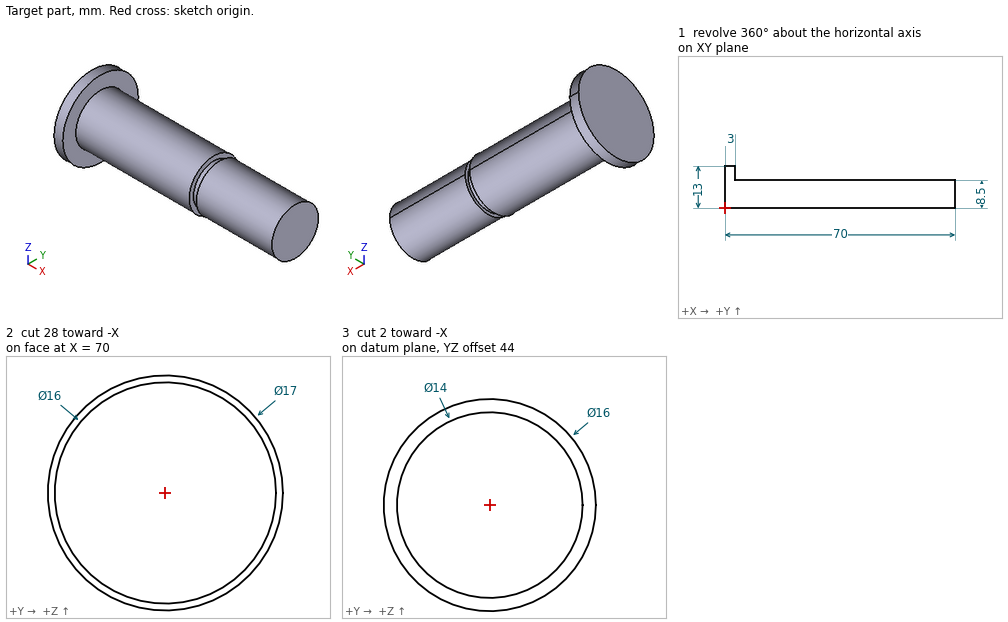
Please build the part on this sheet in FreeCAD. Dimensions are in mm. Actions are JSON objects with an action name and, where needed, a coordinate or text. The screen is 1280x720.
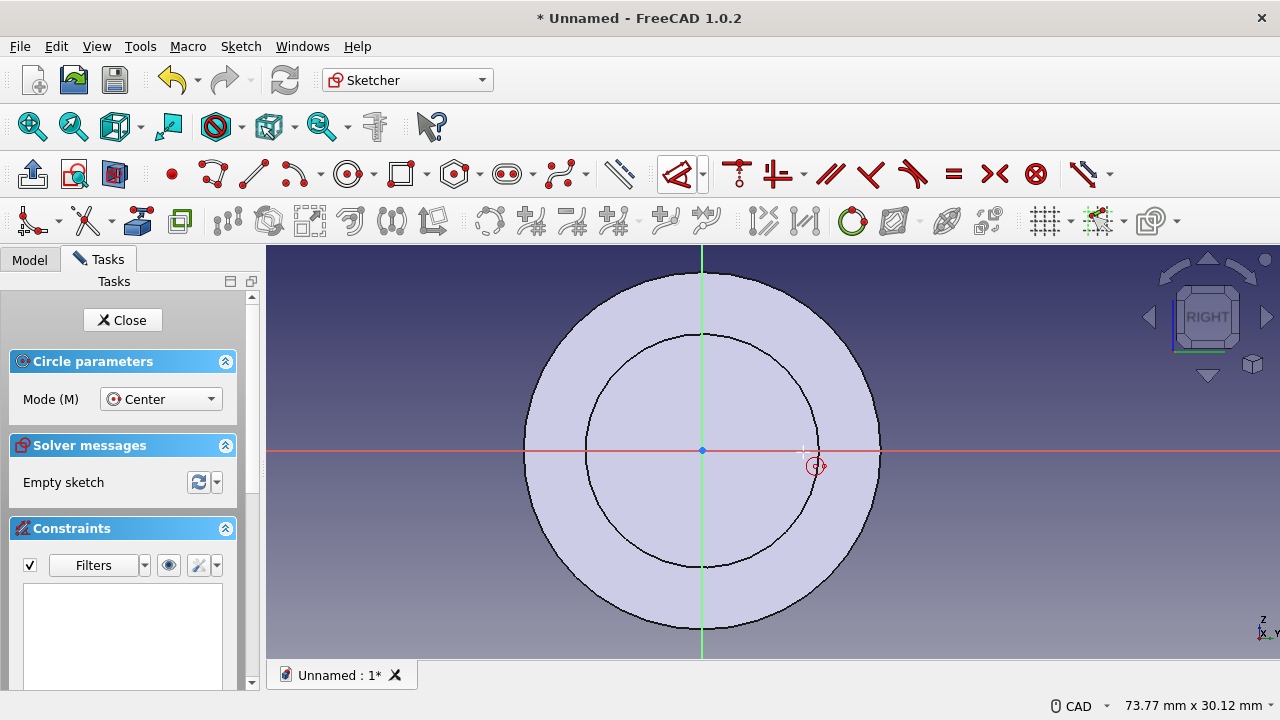
{"action": "left_click", "coordinate": [702, 451]}
{"action": "mouse_move", "coordinate": [785, 368]}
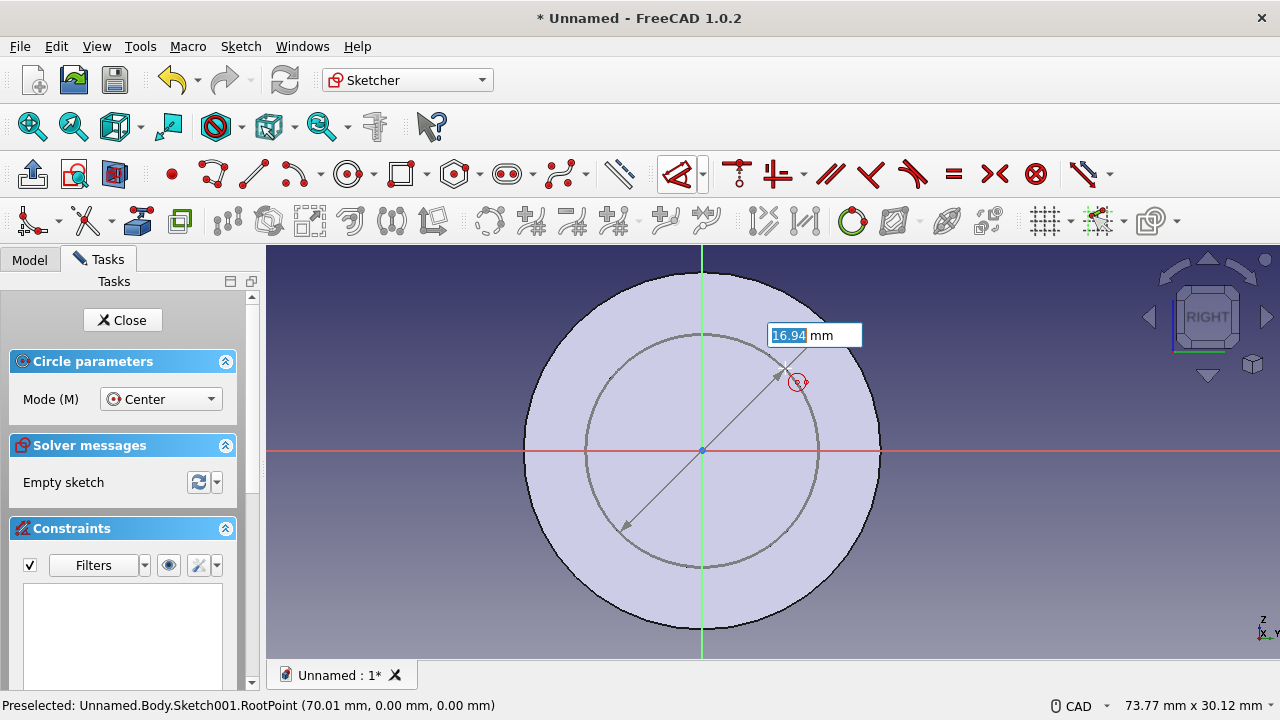
{"action": "type", "text": "17"}
{"action": "key", "text": "Return"}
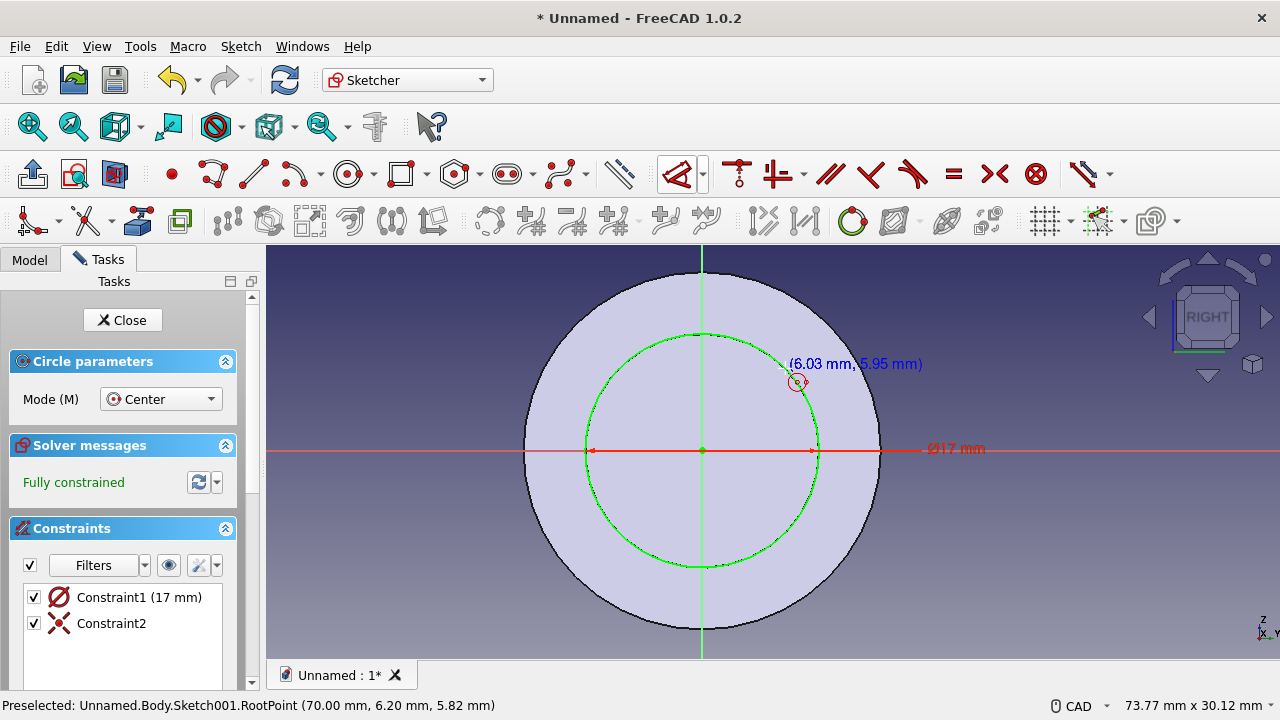
{"action": "left_click", "coordinate": [702, 451]}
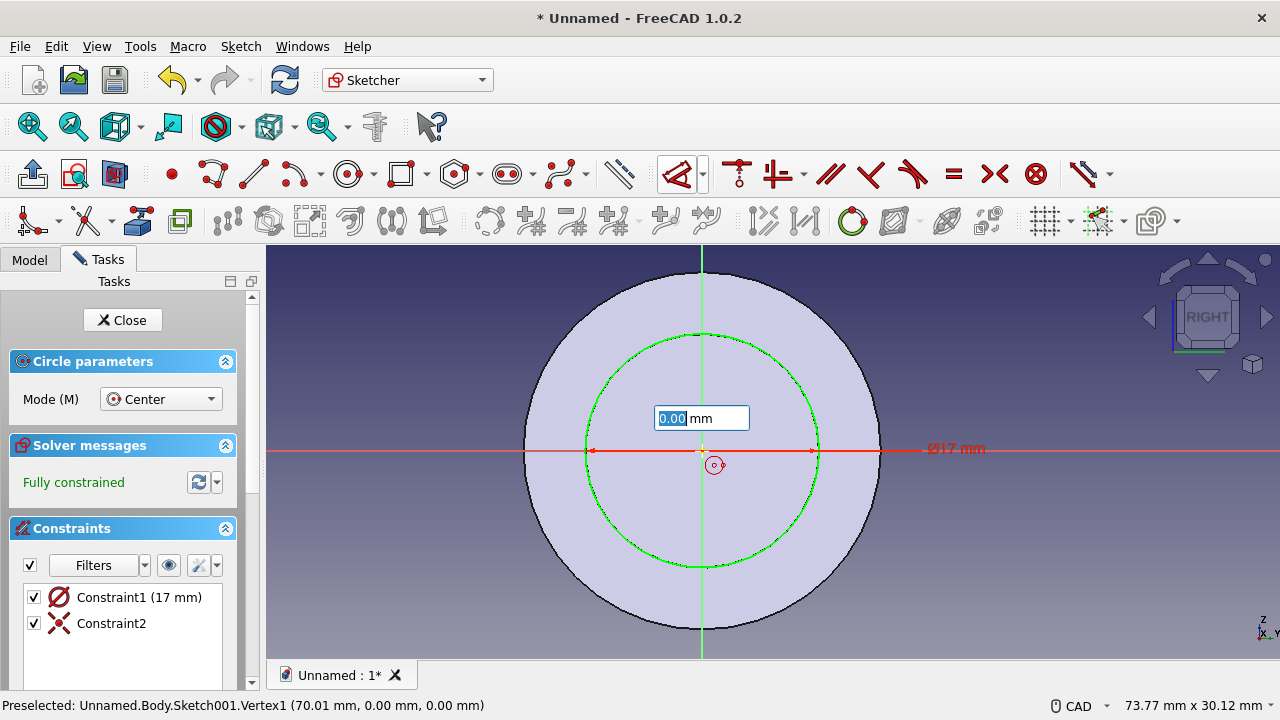
{"action": "scroll", "coordinate": [780, 373], "scroll_direction": "up", "scroll_amount": 5}
{"action": "mouse_move", "coordinate": [779, 373]}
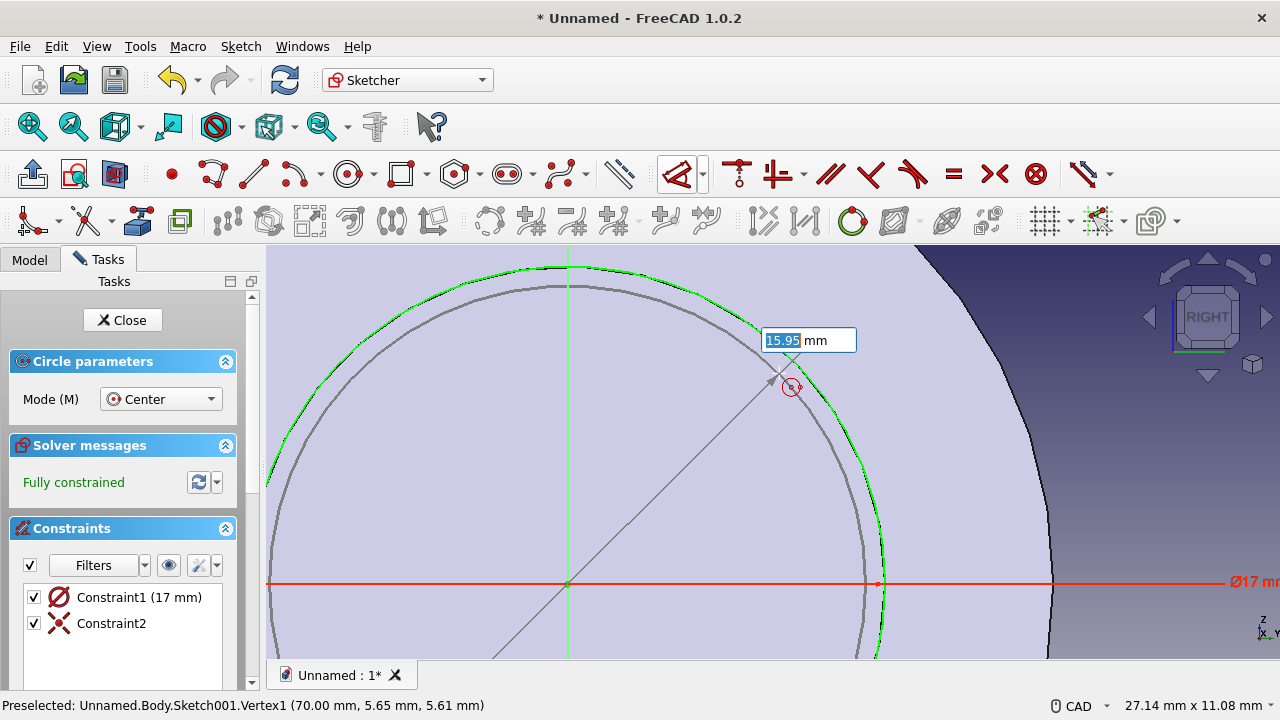
{"action": "type", "text": "16"}
{"action": "key", "text": "Return"}
{"action": "key", "text": "Escape"}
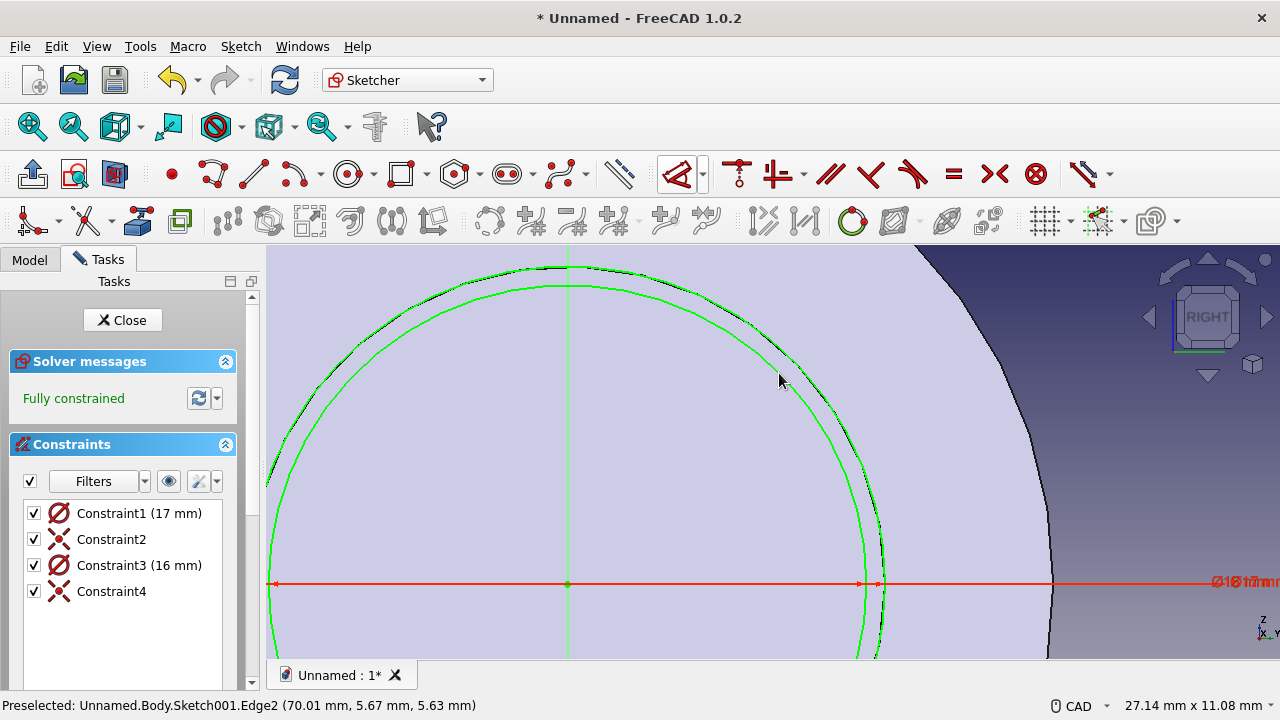
{"action": "left_click", "coordinate": [123, 320]}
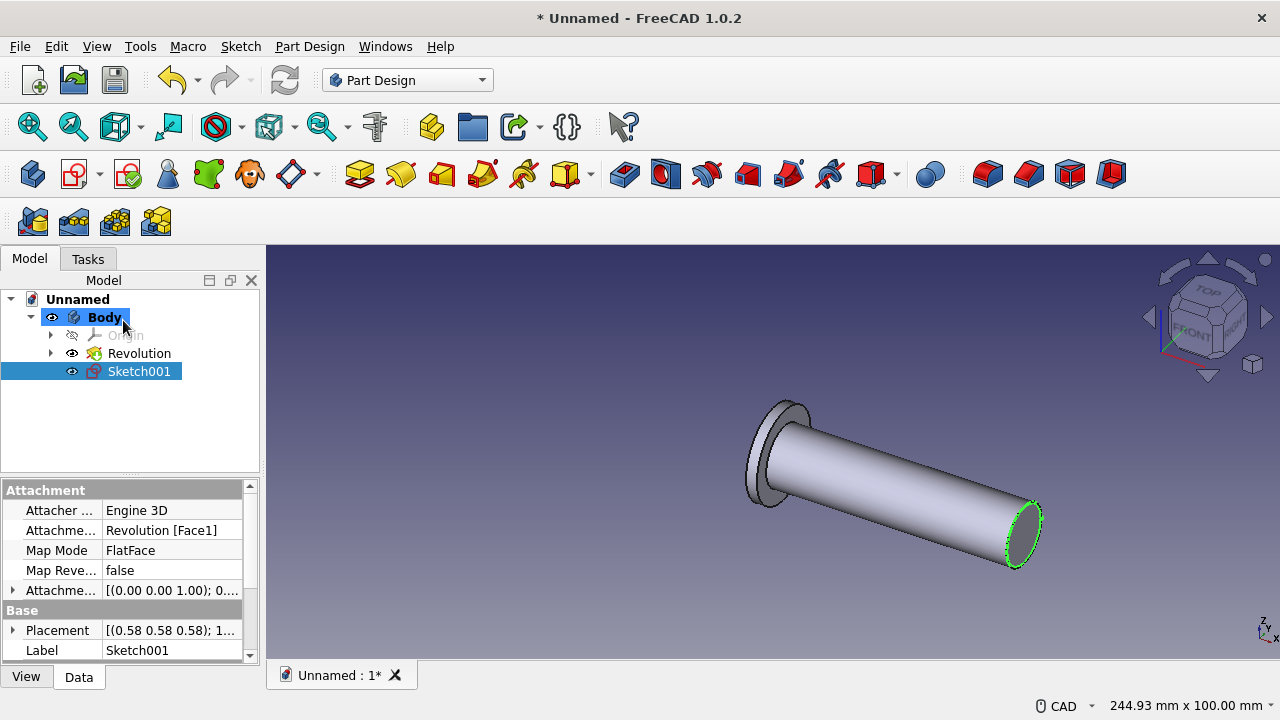
{"action": "left_click", "coordinate": [625, 174]}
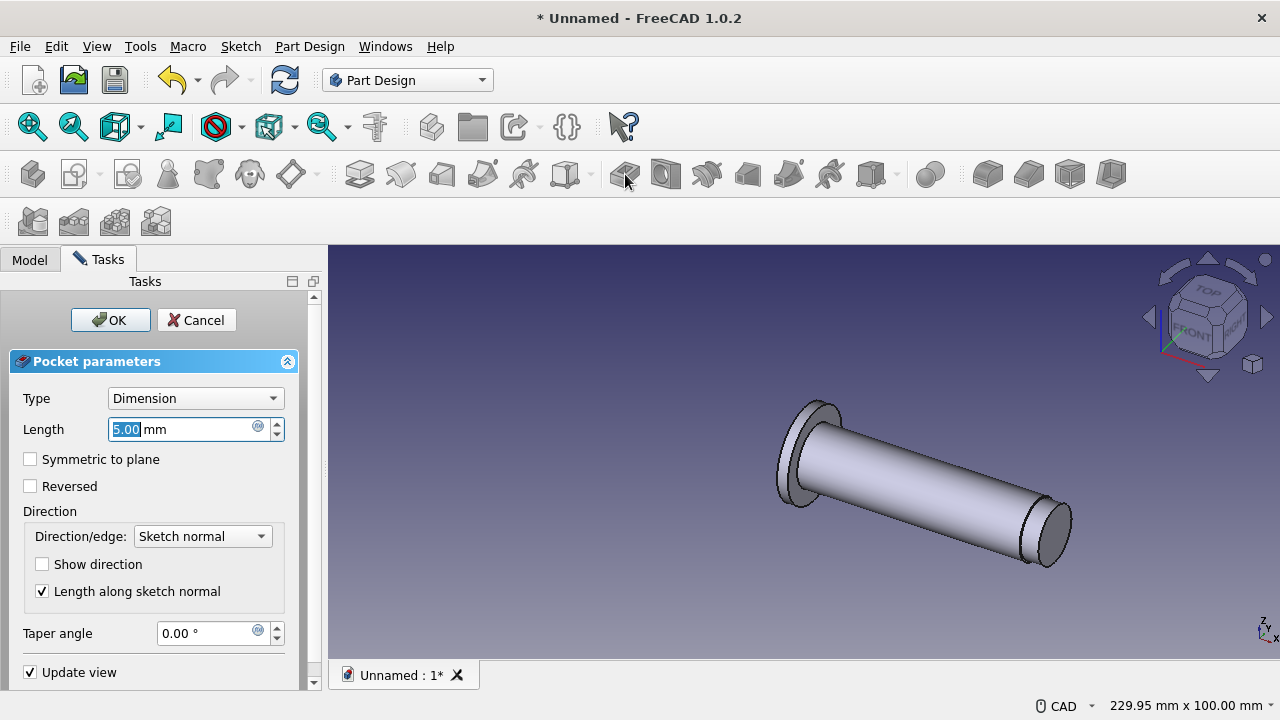
{"action": "type", "text": "28"}
{"action": "key", "text": "Tab"}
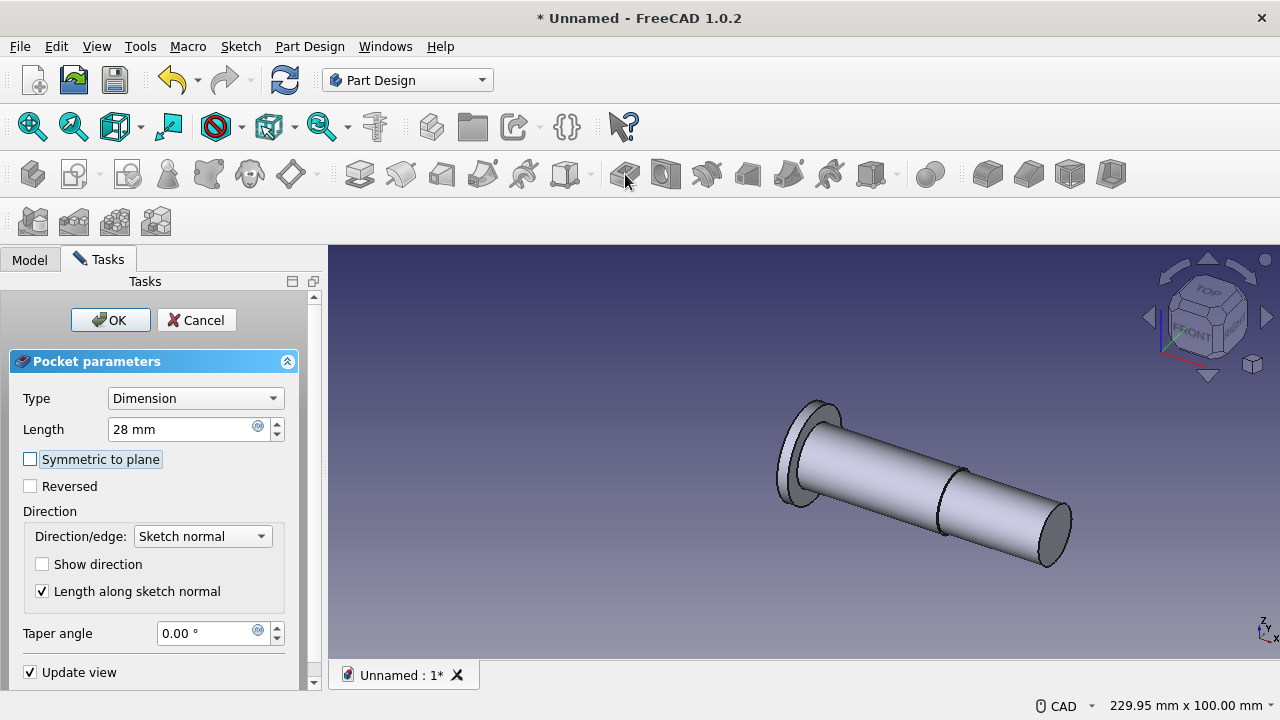
{"action": "left_click", "coordinate": [111, 320]}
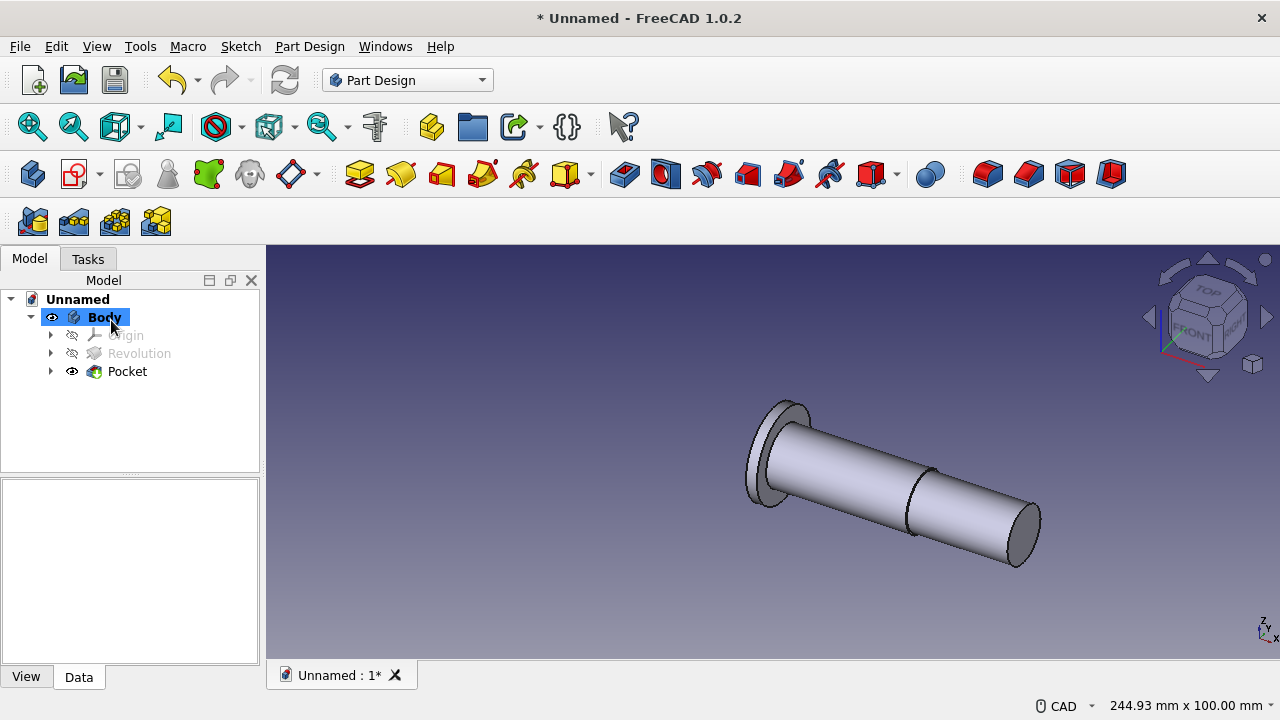
{"action": "left_click", "coordinate": [51, 335]}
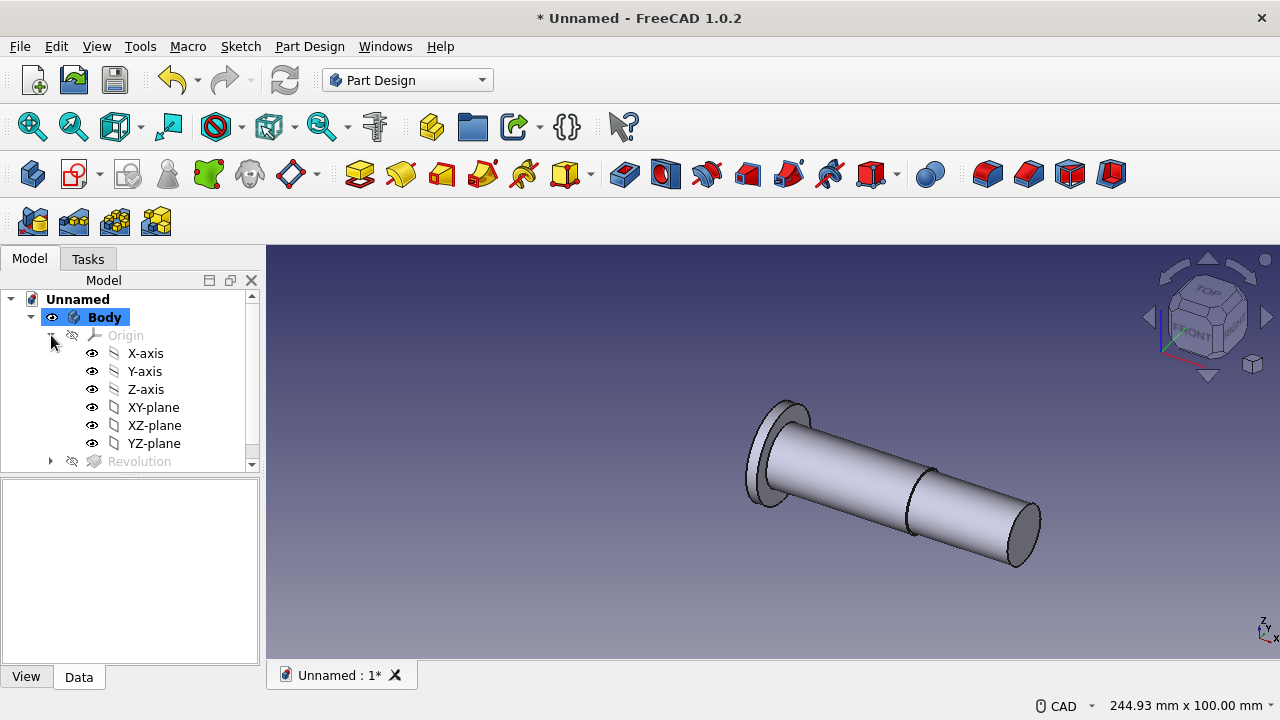
{"action": "left_click", "coordinate": [137, 443]}